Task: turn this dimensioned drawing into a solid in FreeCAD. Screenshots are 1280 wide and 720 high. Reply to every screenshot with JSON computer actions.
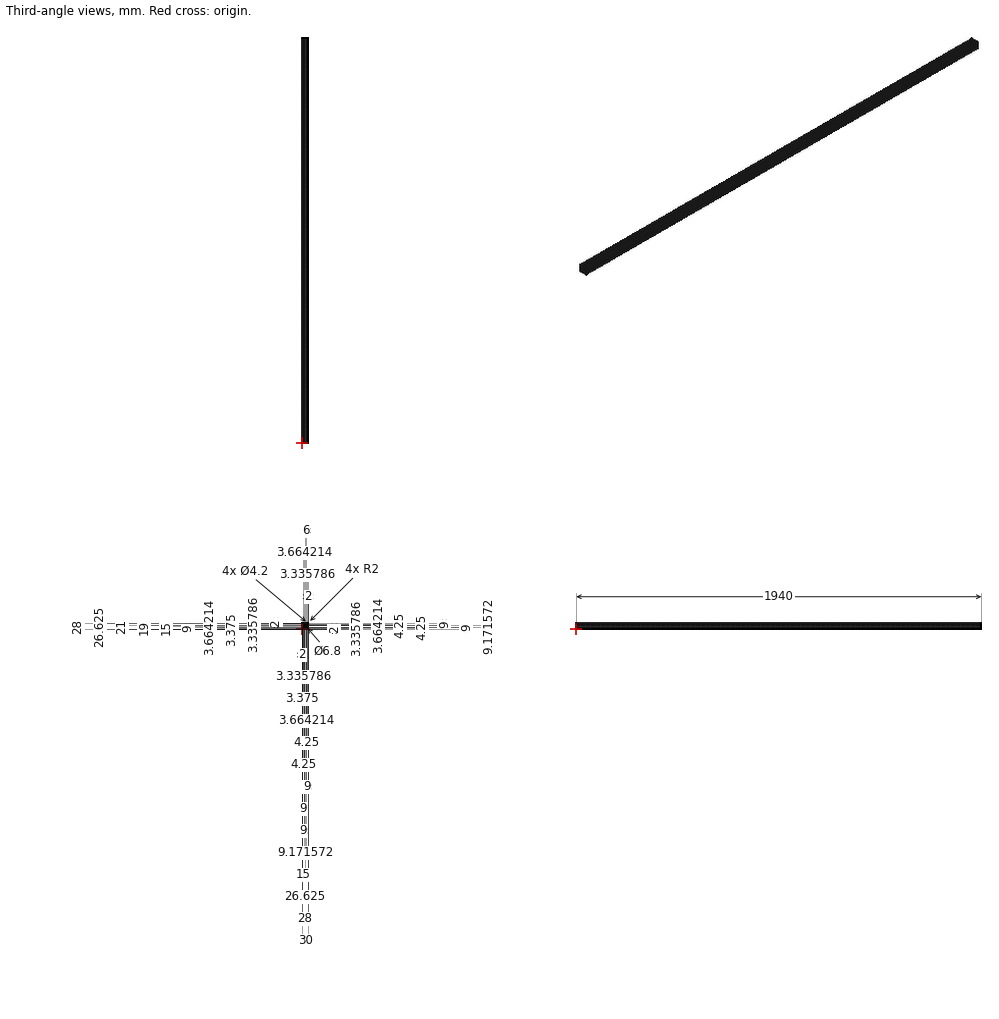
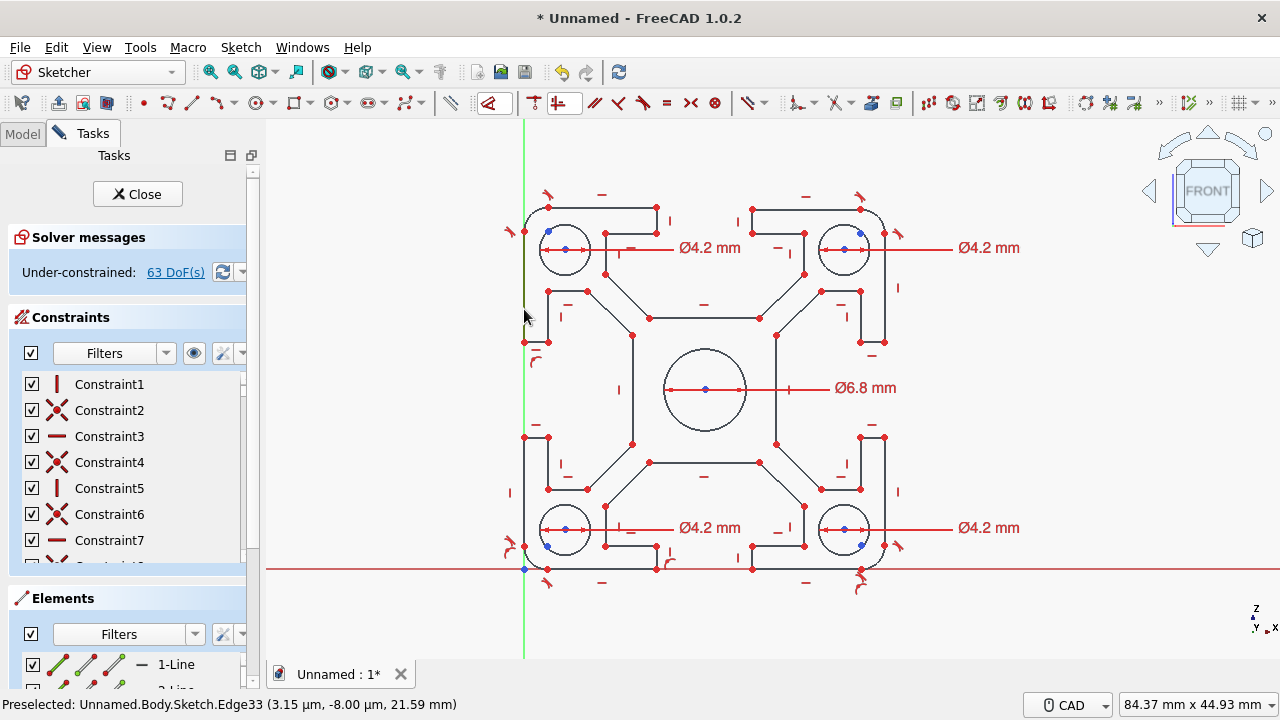
{"action": "key", "text": "v"}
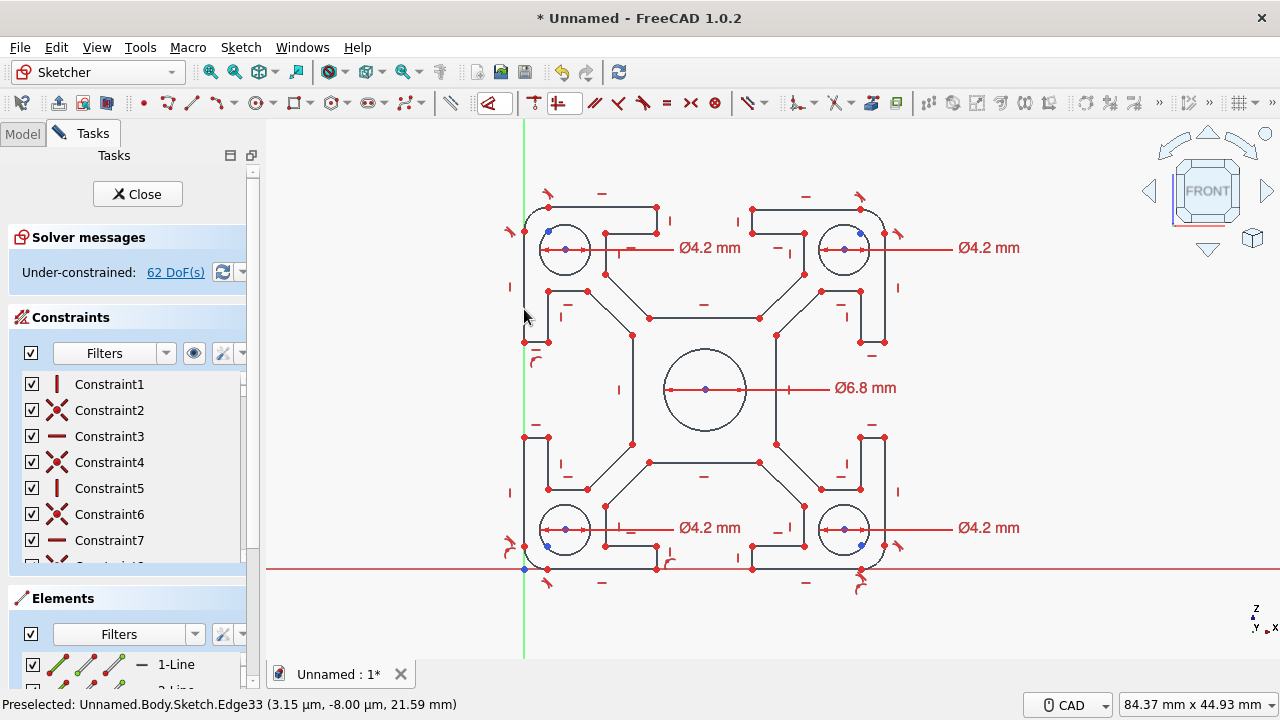
{"action": "scroll", "coordinate": [872, 567], "scroll_direction": "up", "scroll_amount": 2}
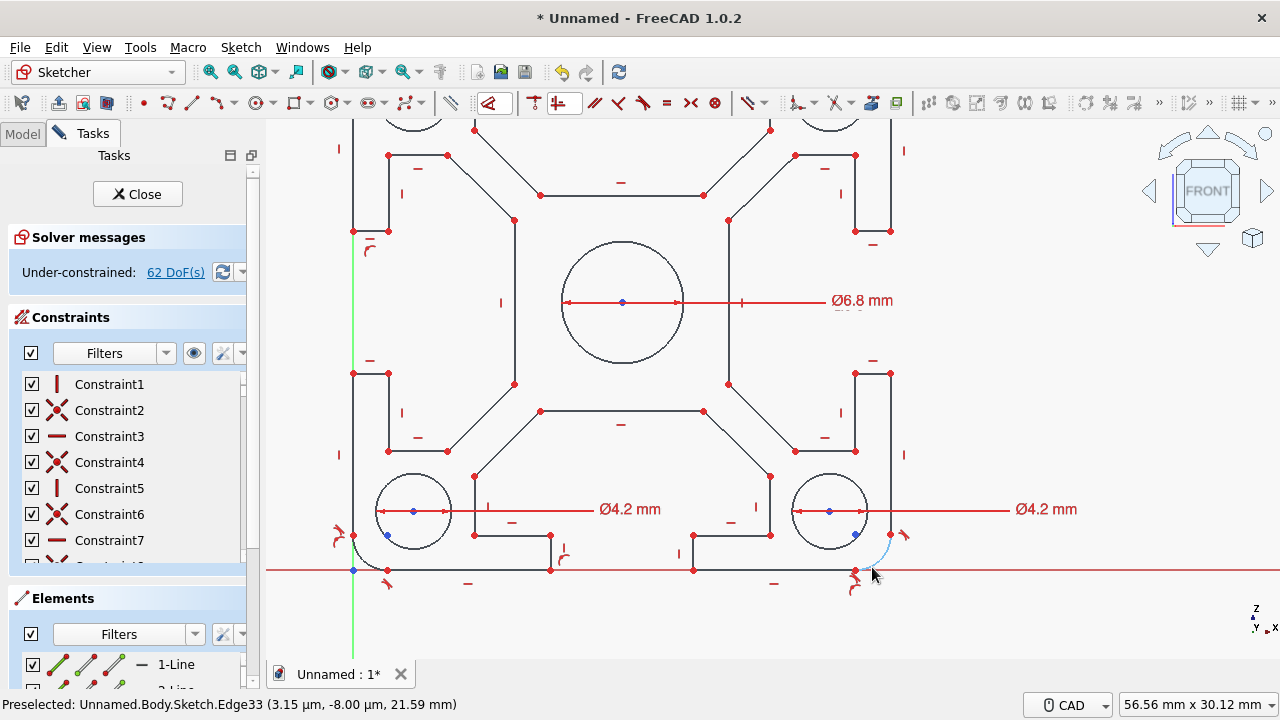
{"action": "left_click", "coordinate": [871, 566]}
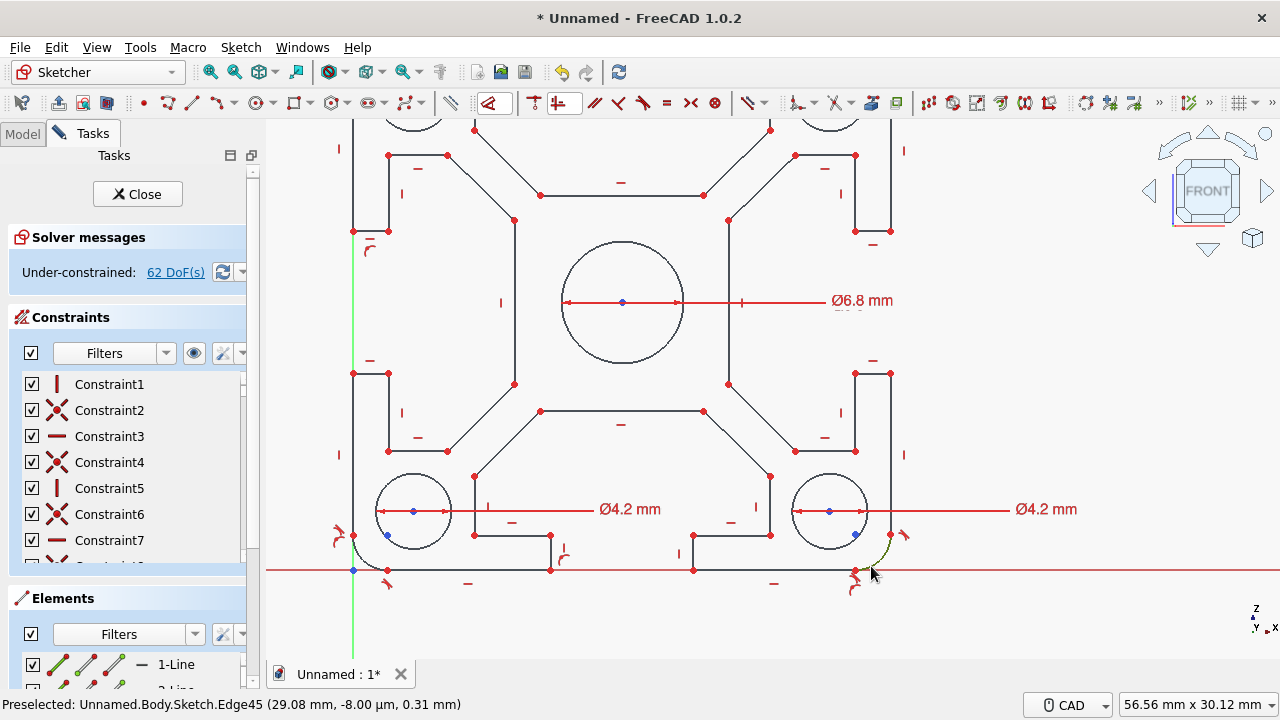
{"action": "left_click", "coordinate": [357, 552]}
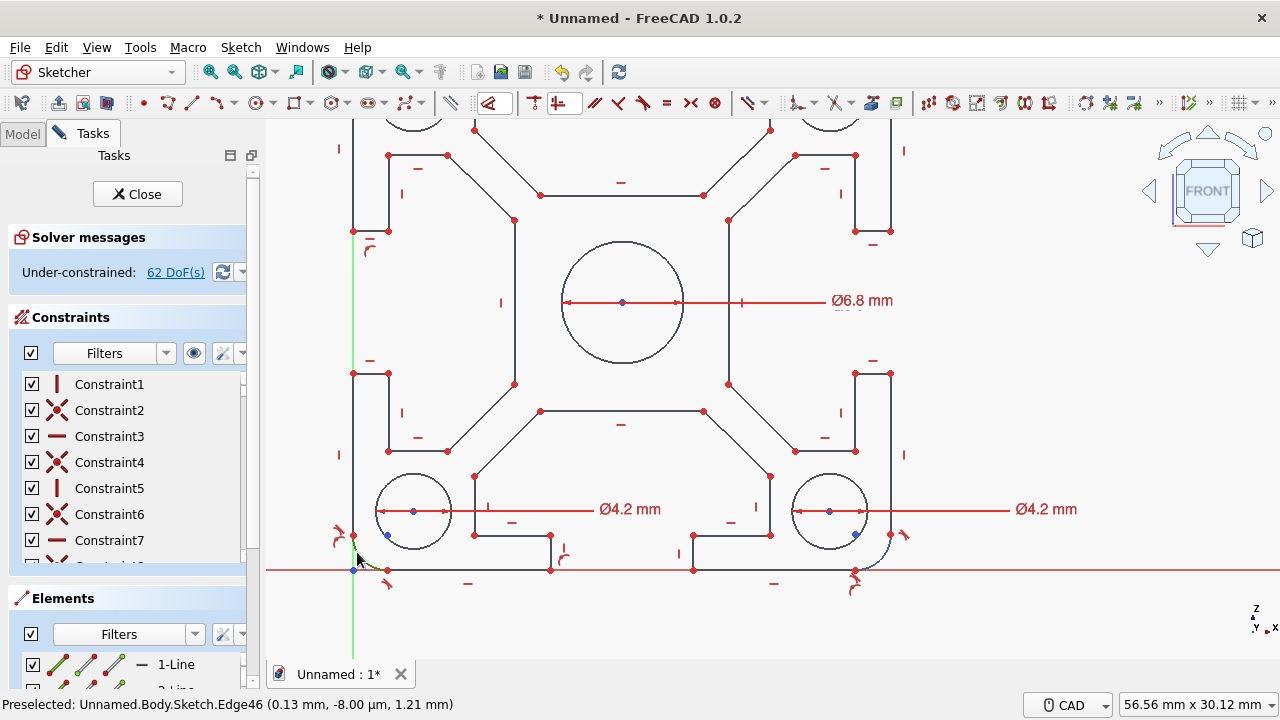
{"action": "scroll", "coordinate": [872, 567], "scroll_direction": "down", "scroll_amount": 2}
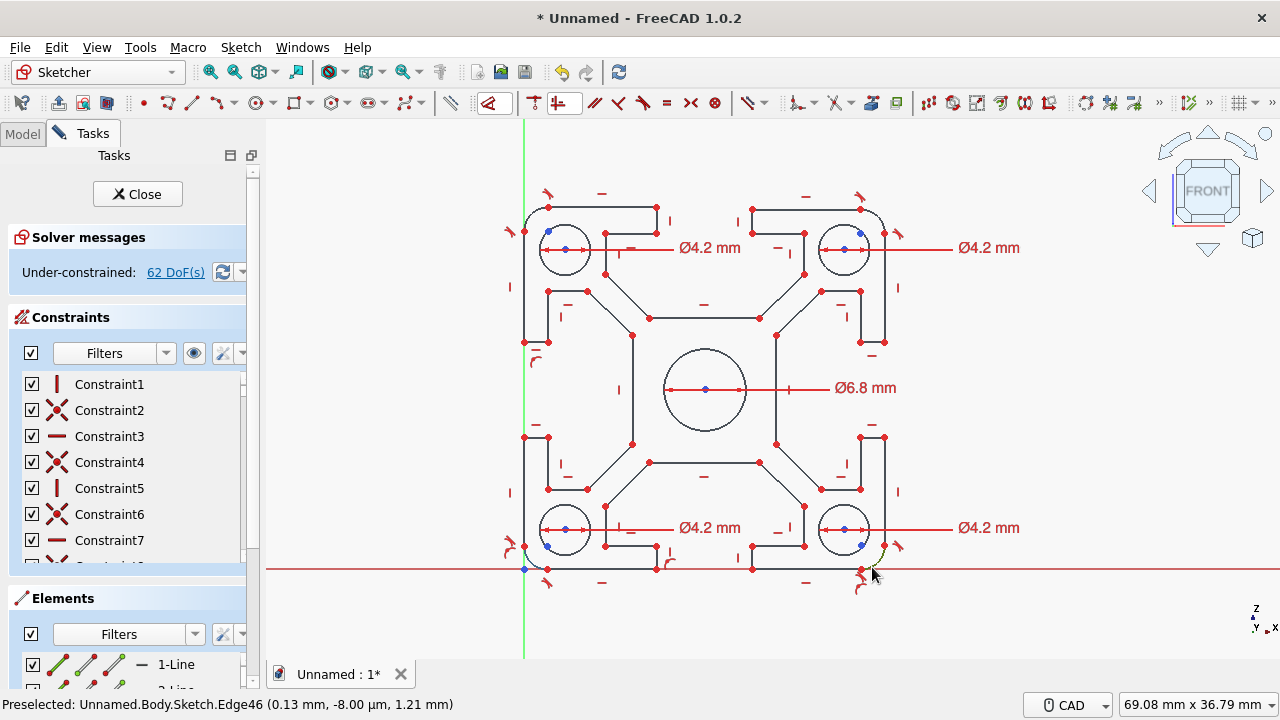
{"action": "scroll", "coordinate": [537, 210], "scroll_direction": "up", "scroll_amount": 2}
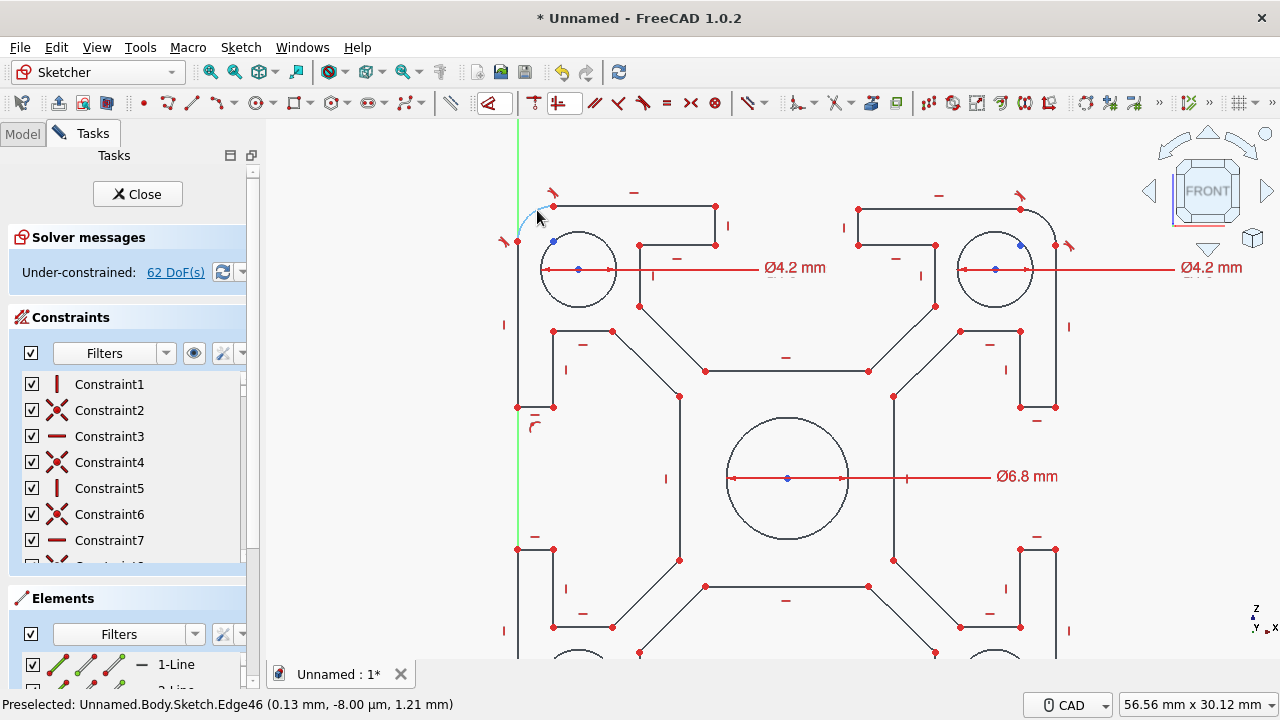
{"action": "left_click", "coordinate": [537, 210]}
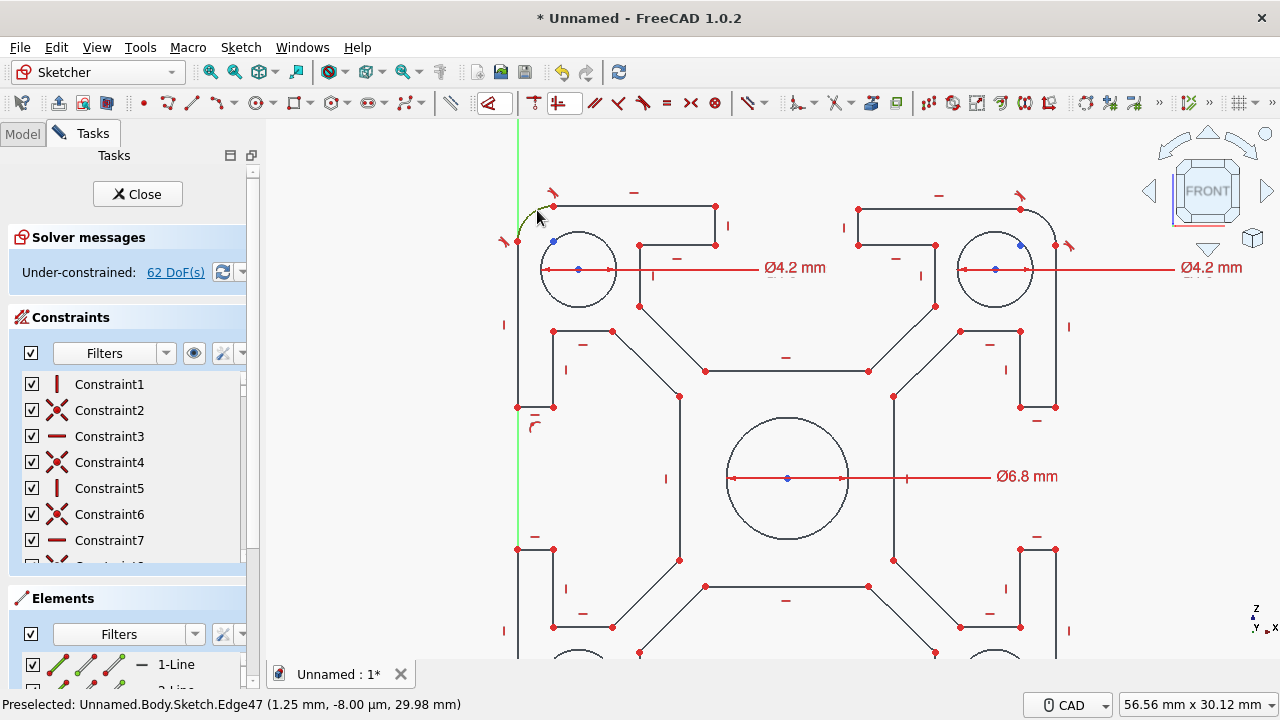
{"action": "left_click", "coordinate": [1052, 229]}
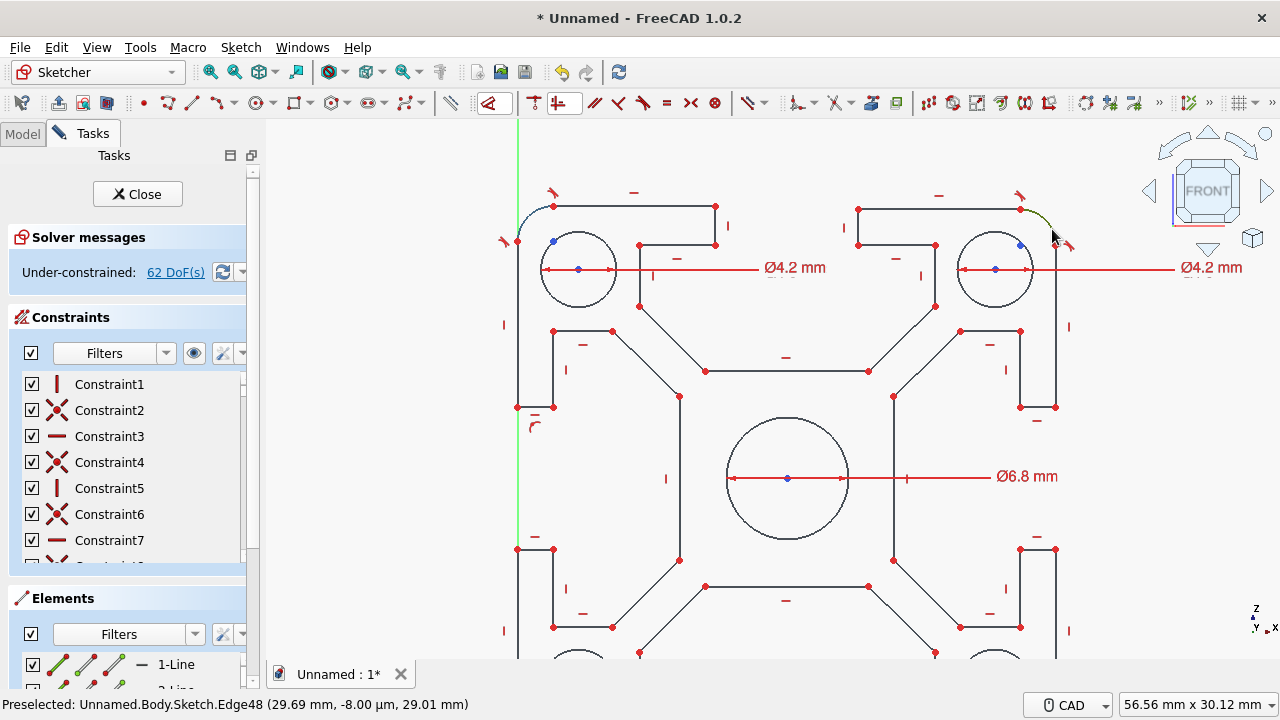
{"action": "left_click", "coordinate": [668, 104]}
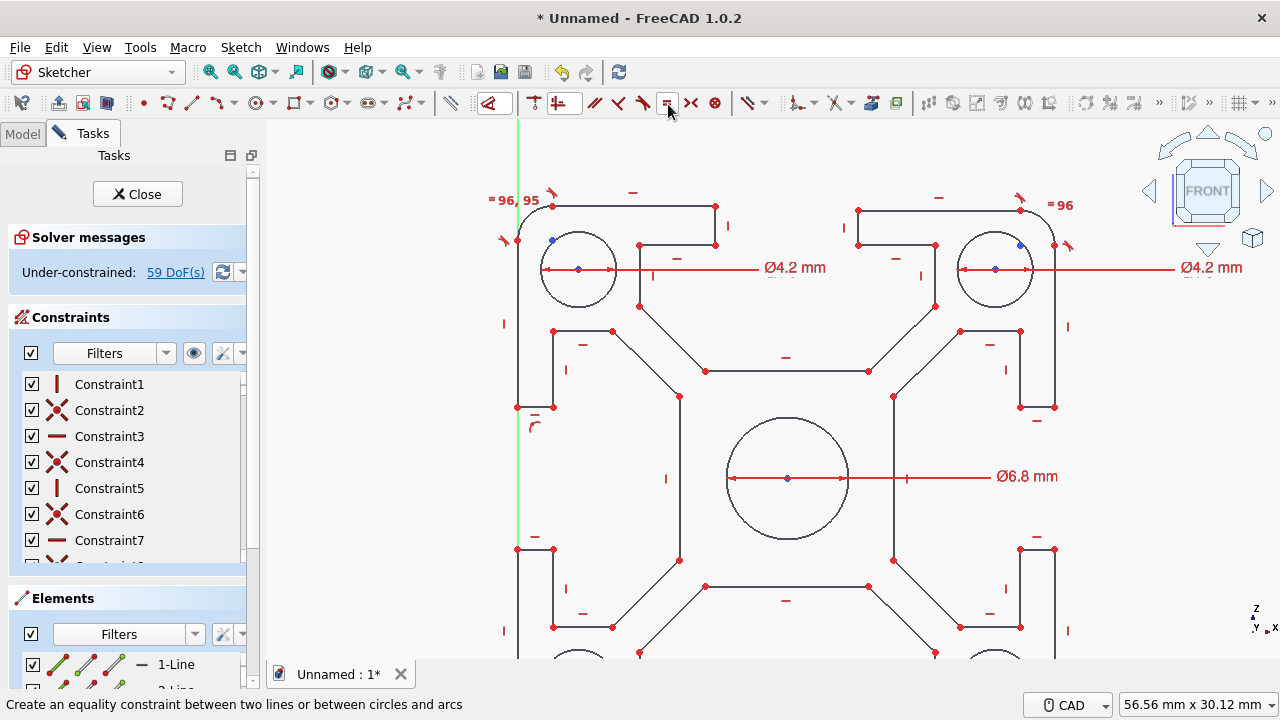
{"action": "left_click", "coordinate": [488, 104]}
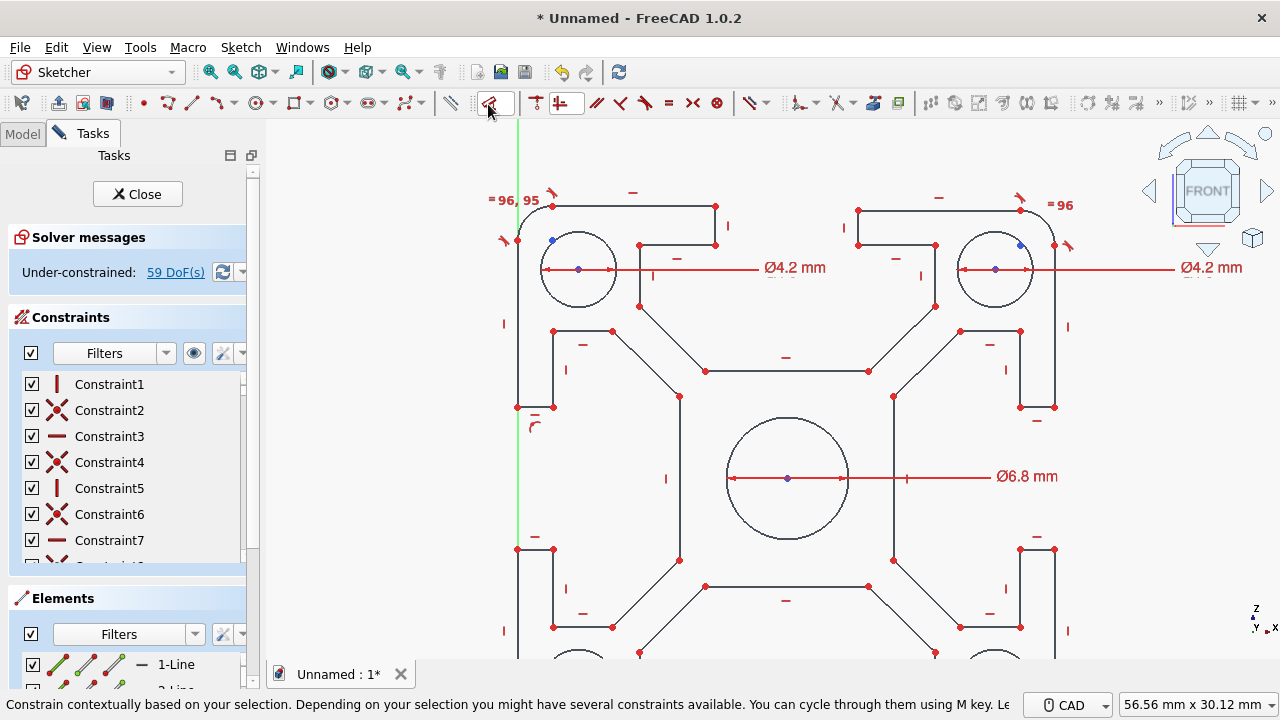
{"action": "scroll", "coordinate": [537, 210], "scroll_direction": "down", "scroll_amount": 2}